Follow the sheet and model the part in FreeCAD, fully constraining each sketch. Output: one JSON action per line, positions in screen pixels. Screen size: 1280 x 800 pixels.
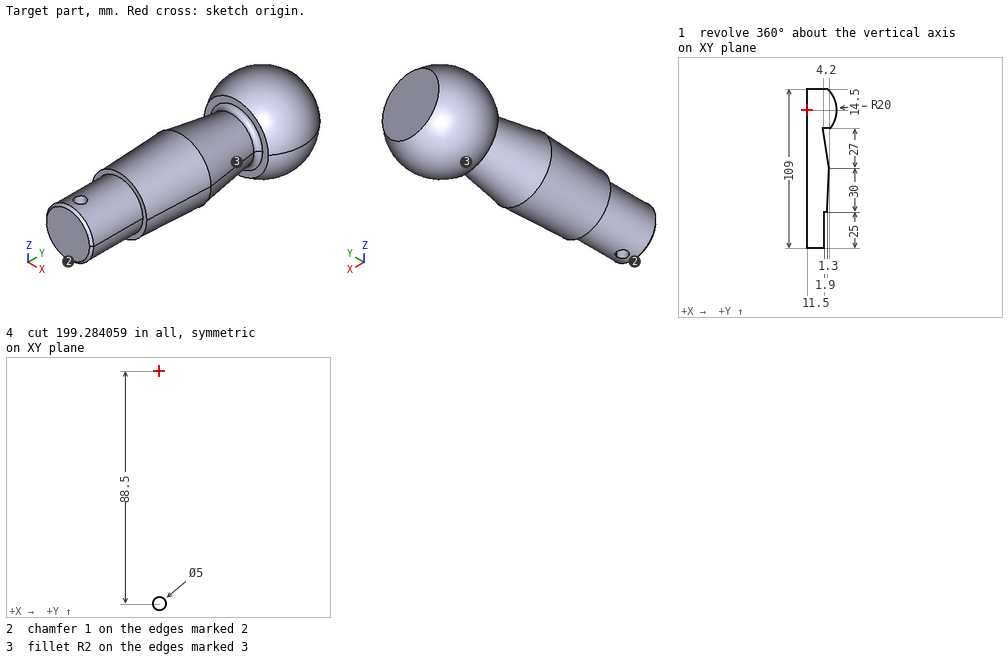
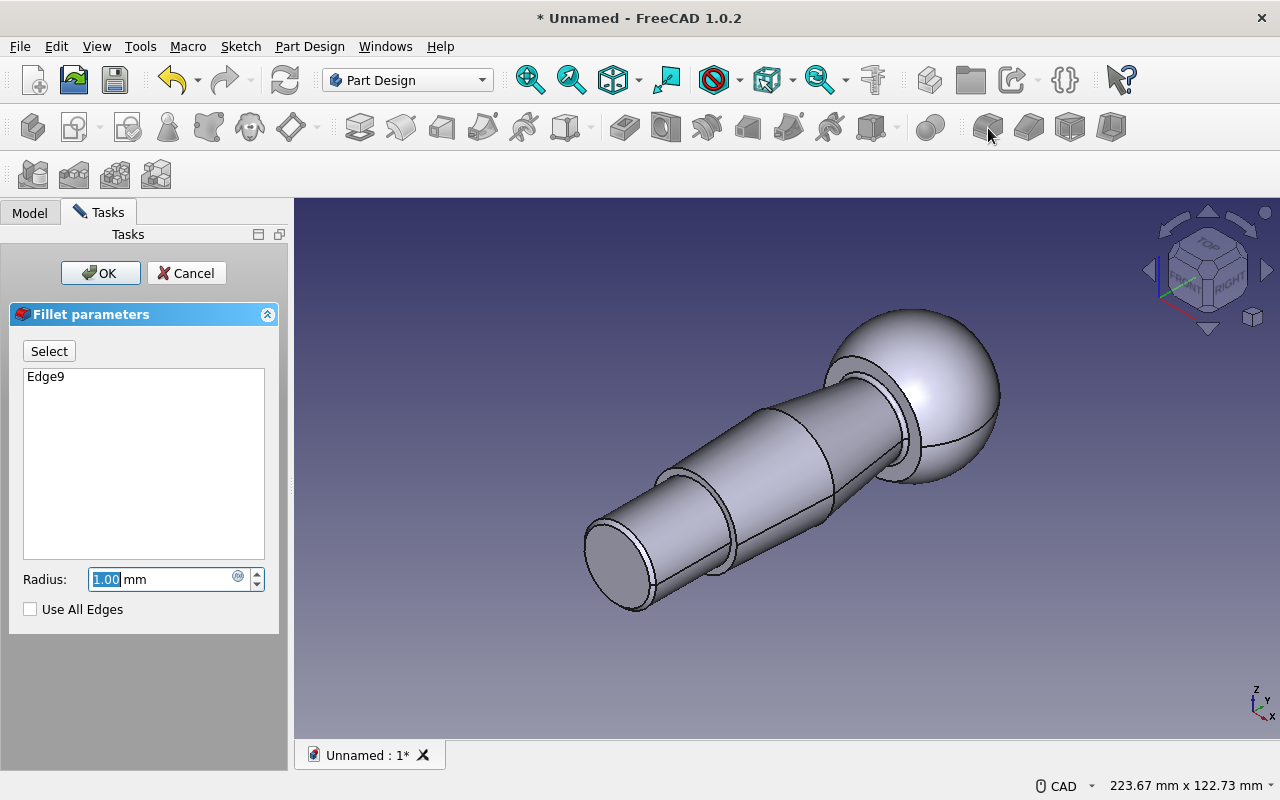
{"action": "type", "text": "2"}
{"action": "key", "text": "Tab"}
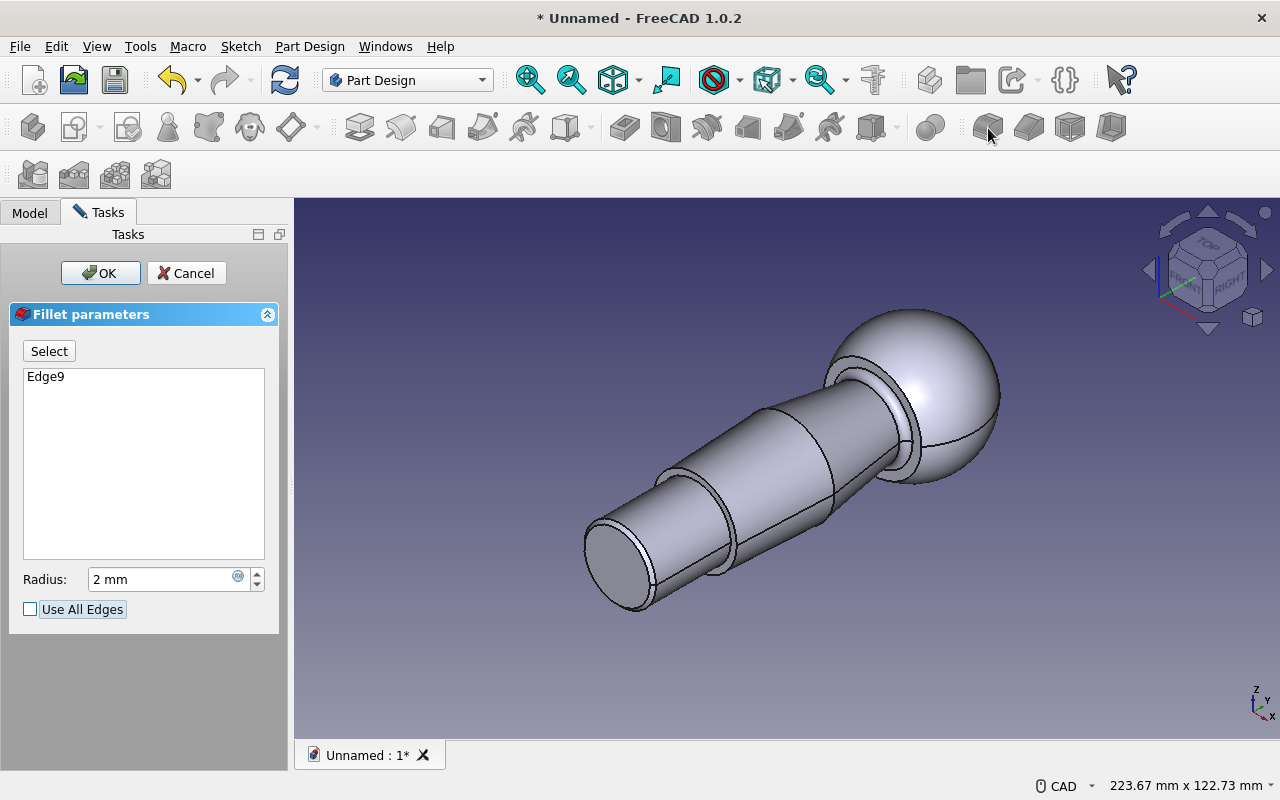
{"action": "left_click", "coordinate": [101, 273]}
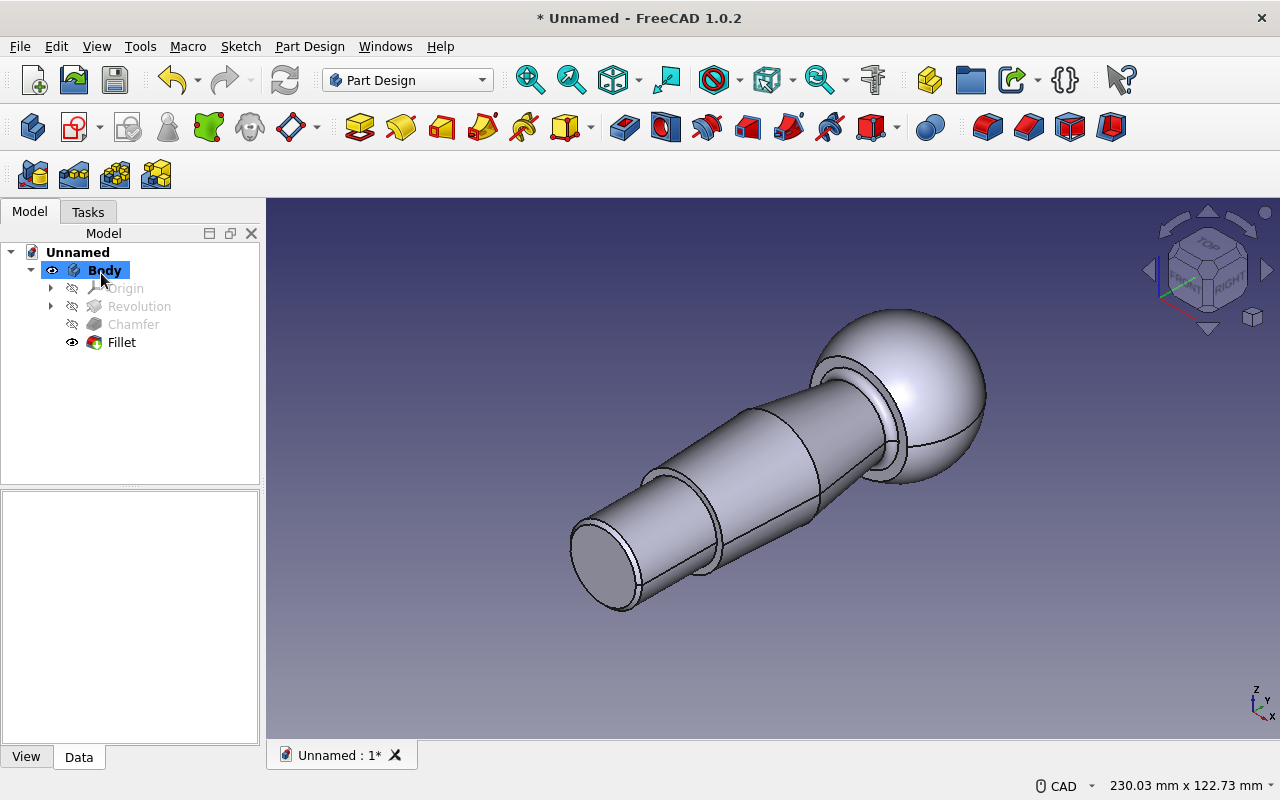
{"action": "left_click", "coordinate": [74, 128]}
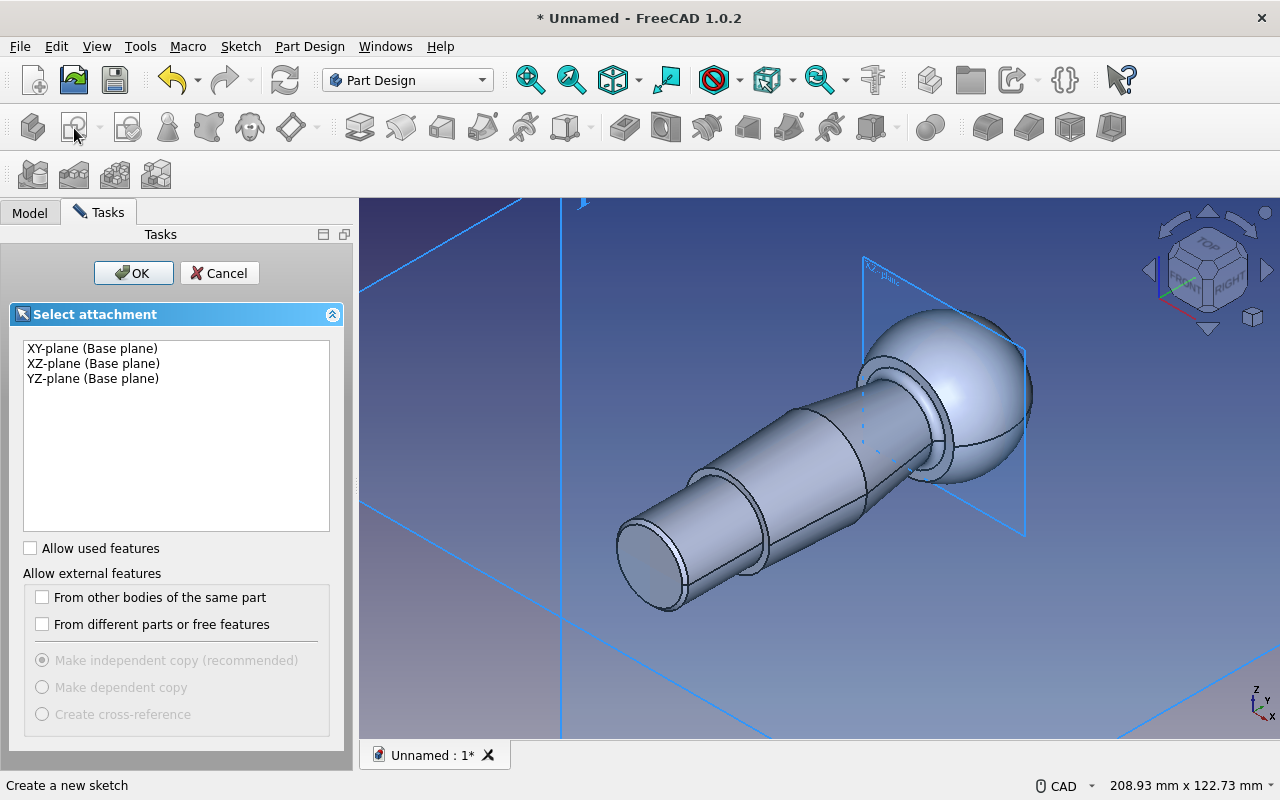
{"action": "left_click", "coordinate": [84, 348]}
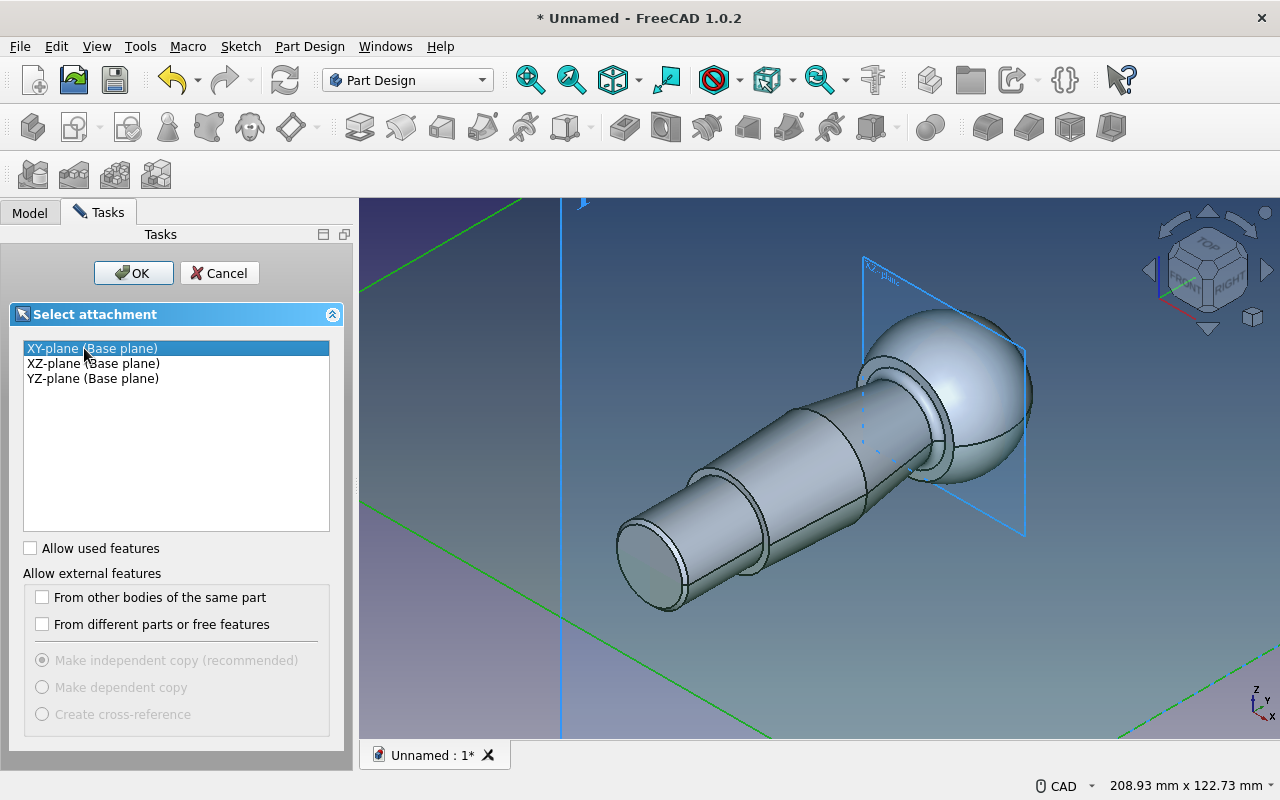
{"action": "left_click", "coordinate": [134, 273]}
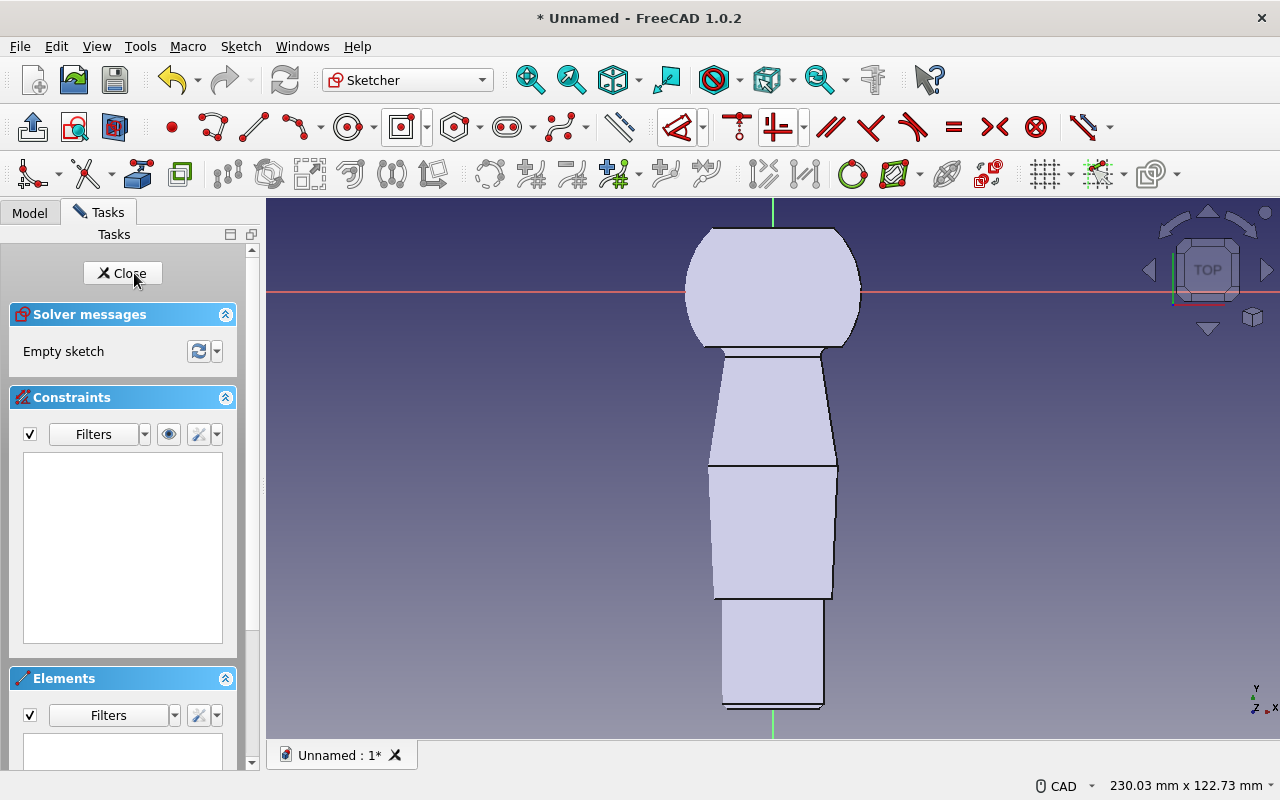
{"action": "left_click", "coordinate": [115, 128]}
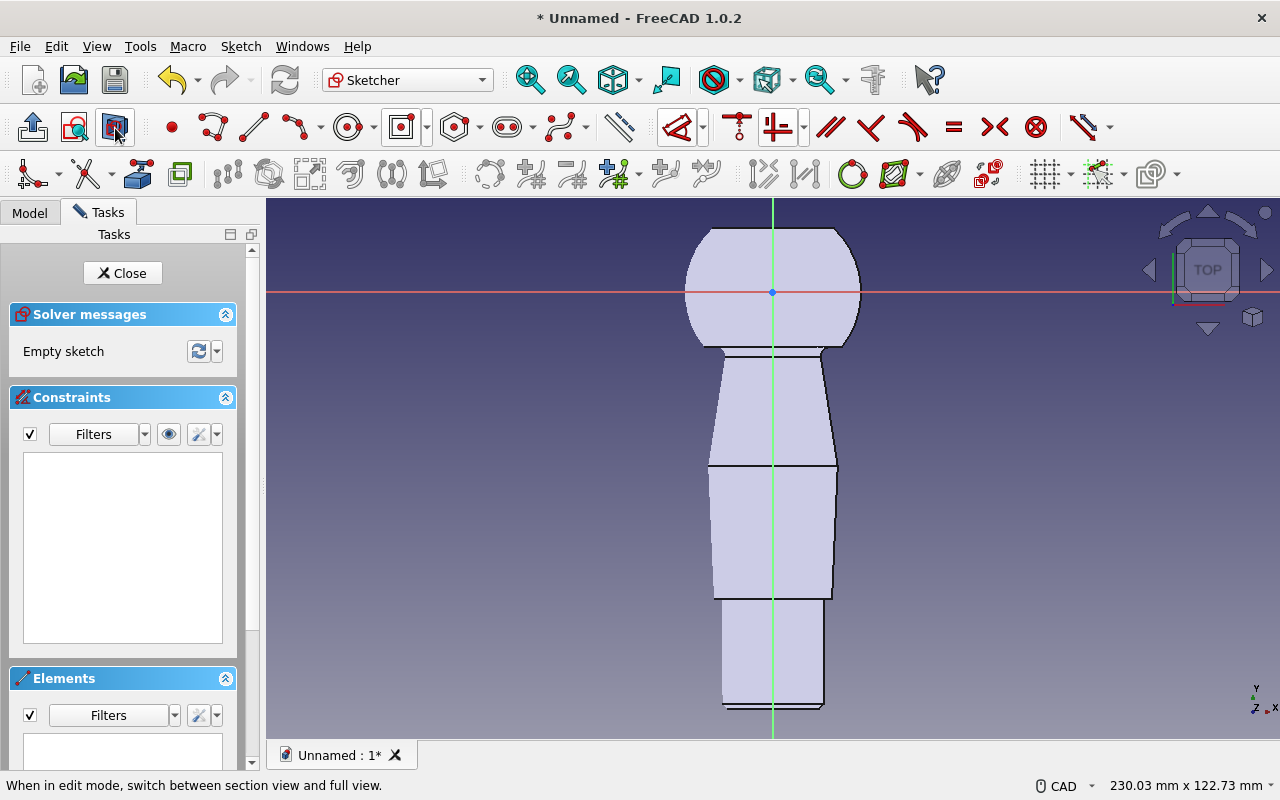
{"action": "scroll", "coordinate": [777, 696], "scroll_direction": "up", "scroll_amount": 14}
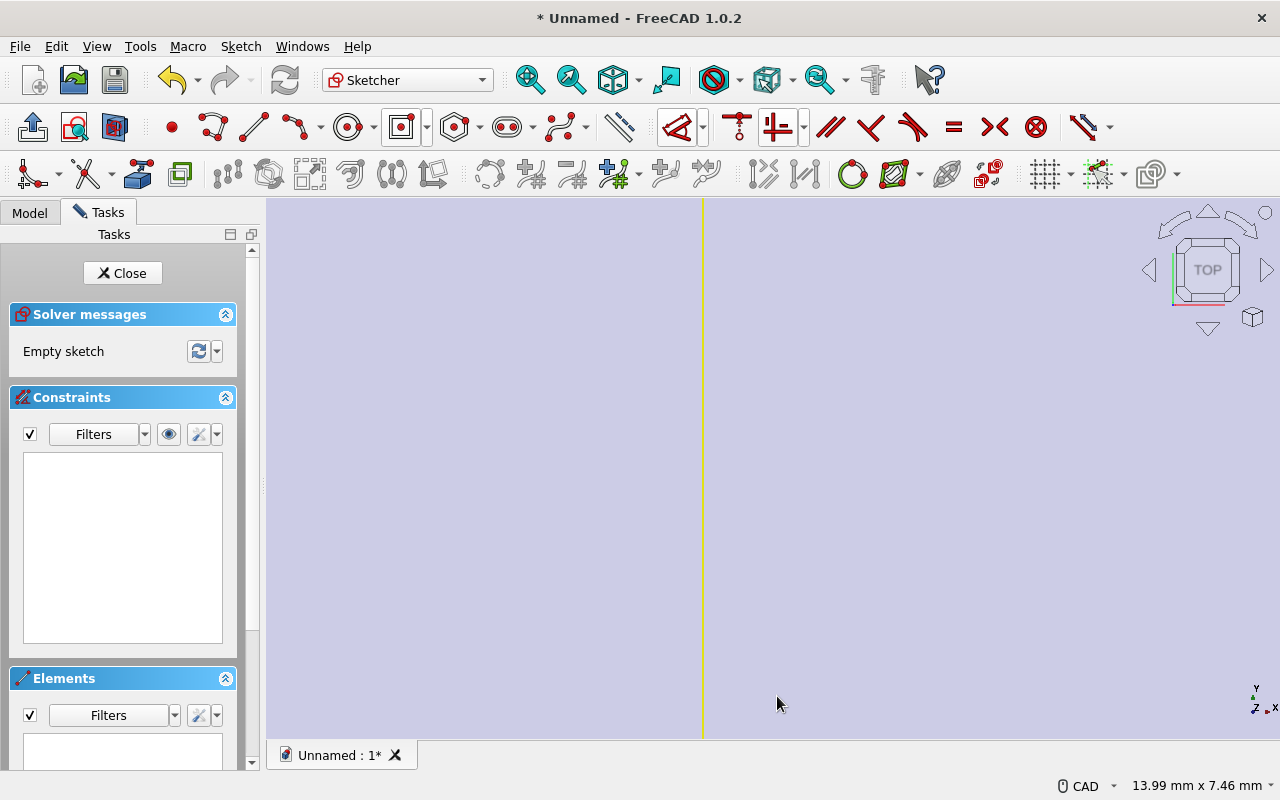
{"action": "left_click", "coordinate": [348, 128]}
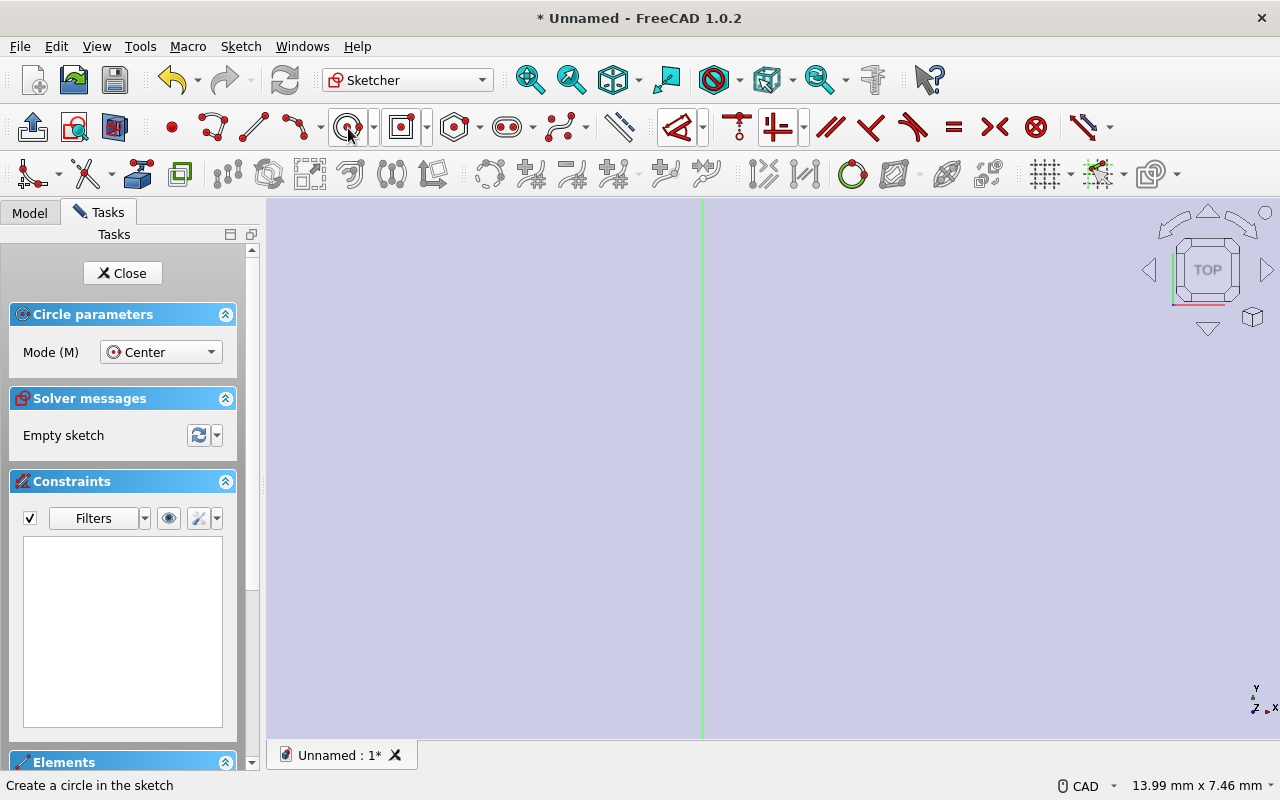
{"action": "left_click", "coordinate": [703, 456]}
{"action": "left_click", "coordinate": [831, 328]}
{"action": "key", "text": "Escape"}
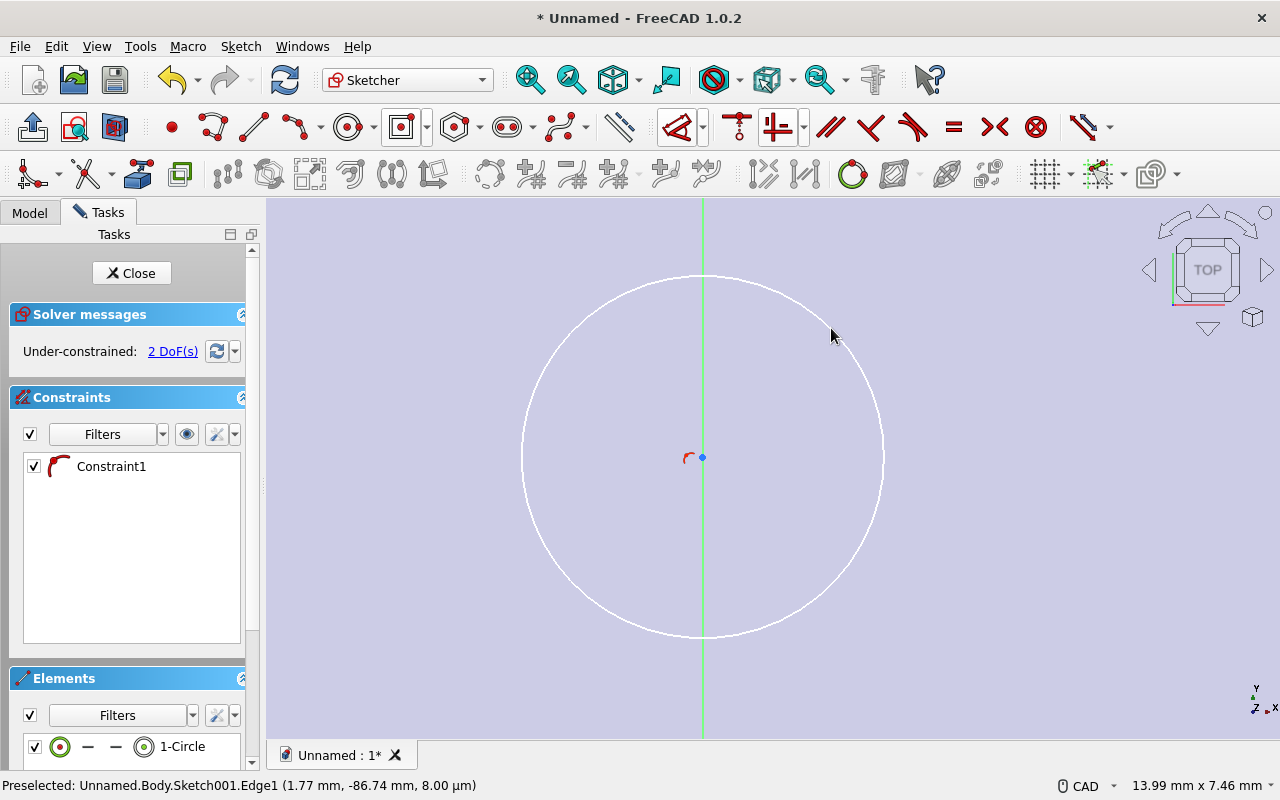
{"action": "left_click", "coordinate": [830, 328]}